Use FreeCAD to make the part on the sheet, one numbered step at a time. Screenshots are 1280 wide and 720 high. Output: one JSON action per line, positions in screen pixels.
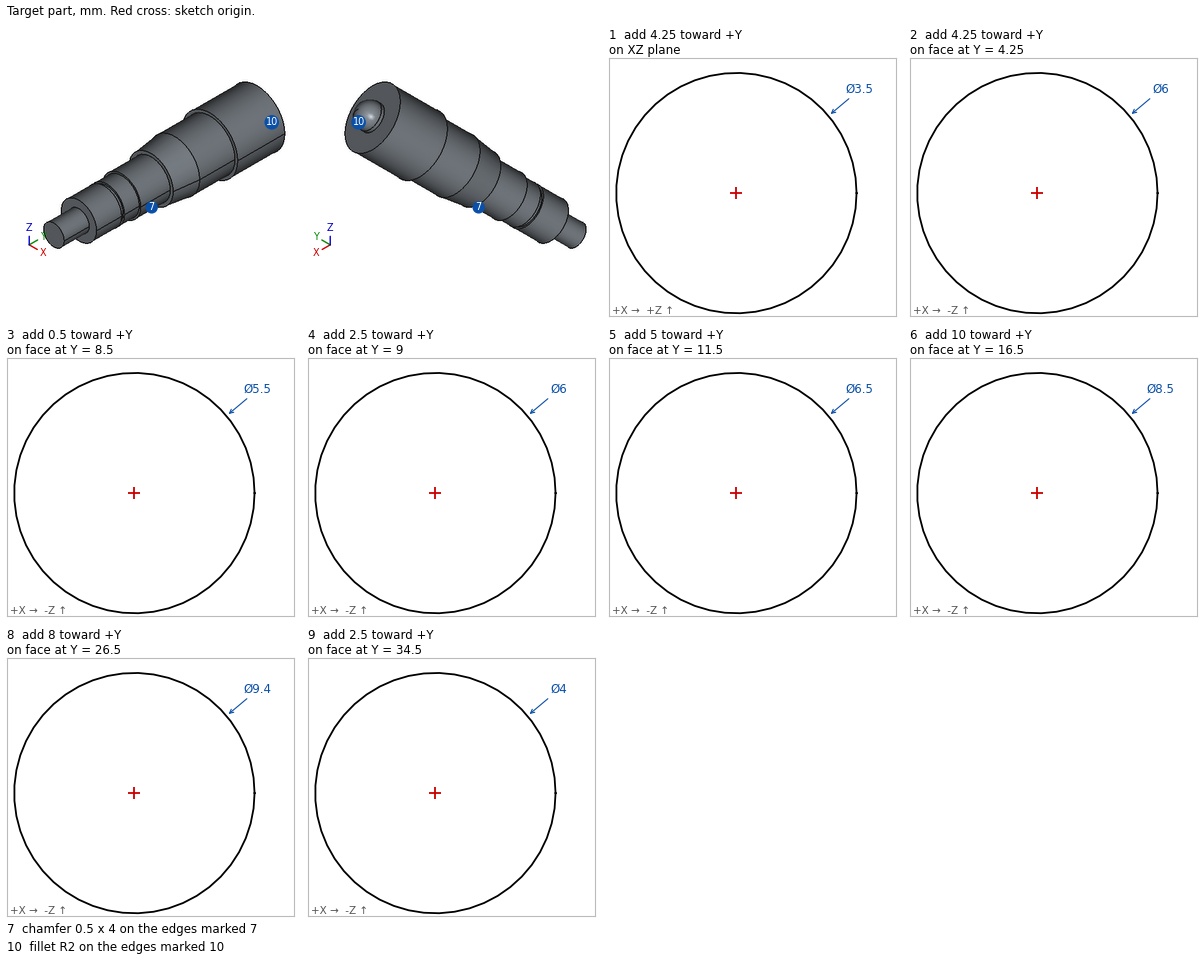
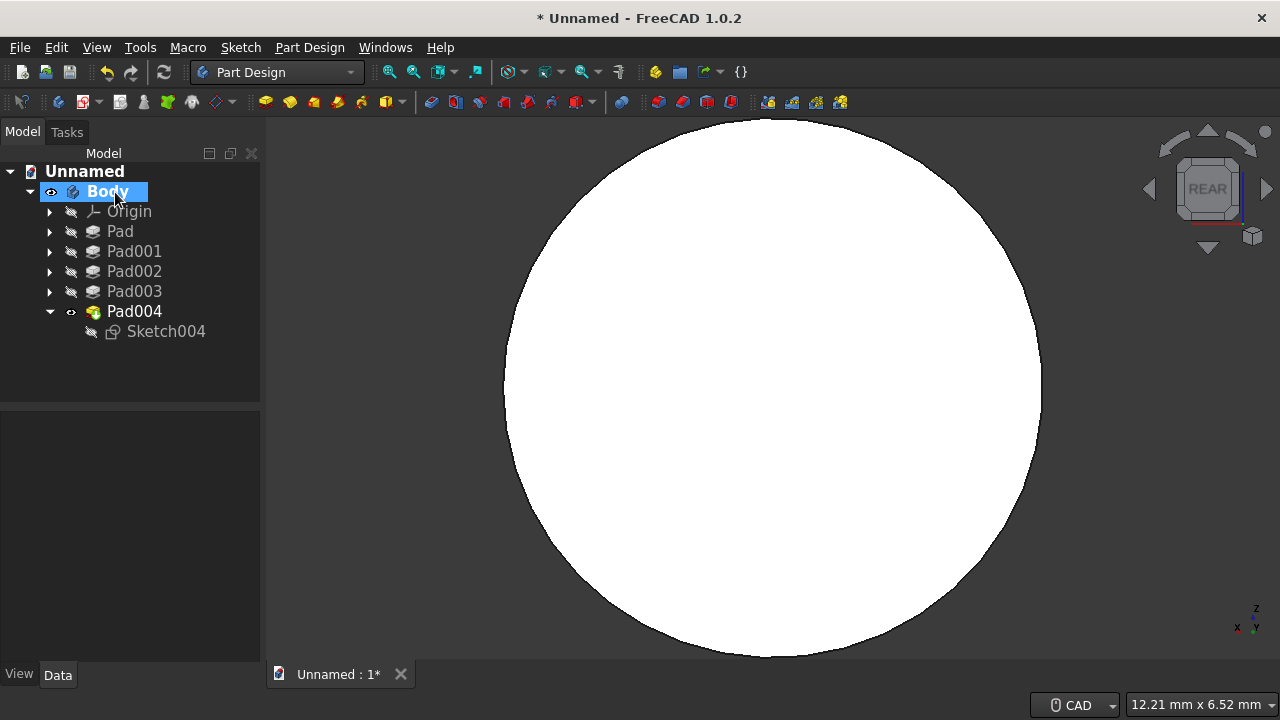
{"action": "left_click", "coordinate": [773, 387]}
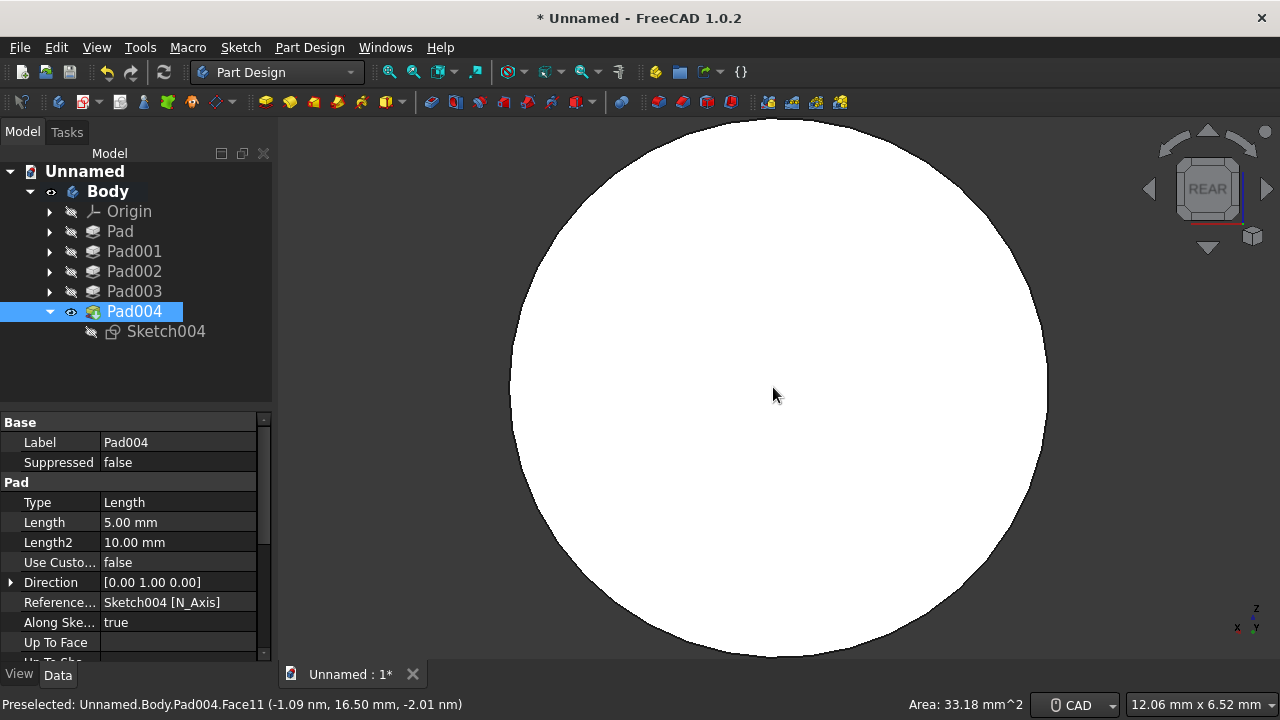
{"action": "left_click", "coordinate": [84, 102]}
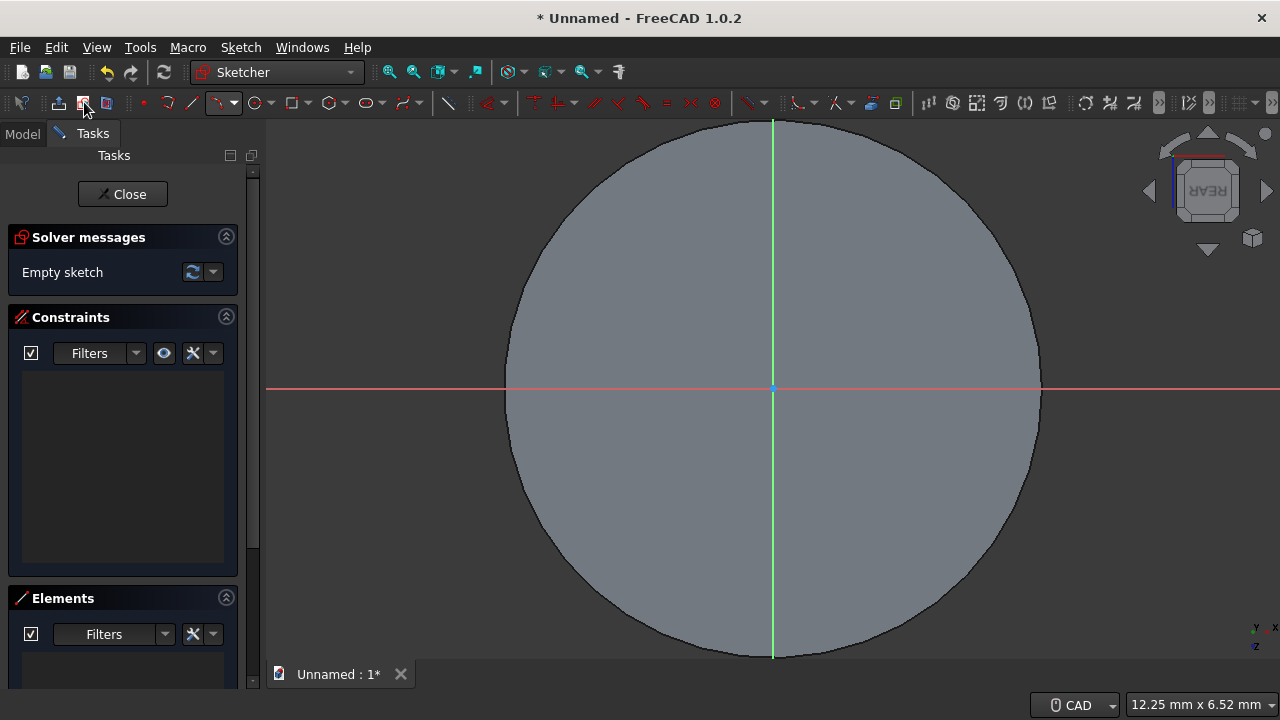
{"action": "scroll", "coordinate": [649, 389], "scroll_direction": "down", "scroll_amount": 4}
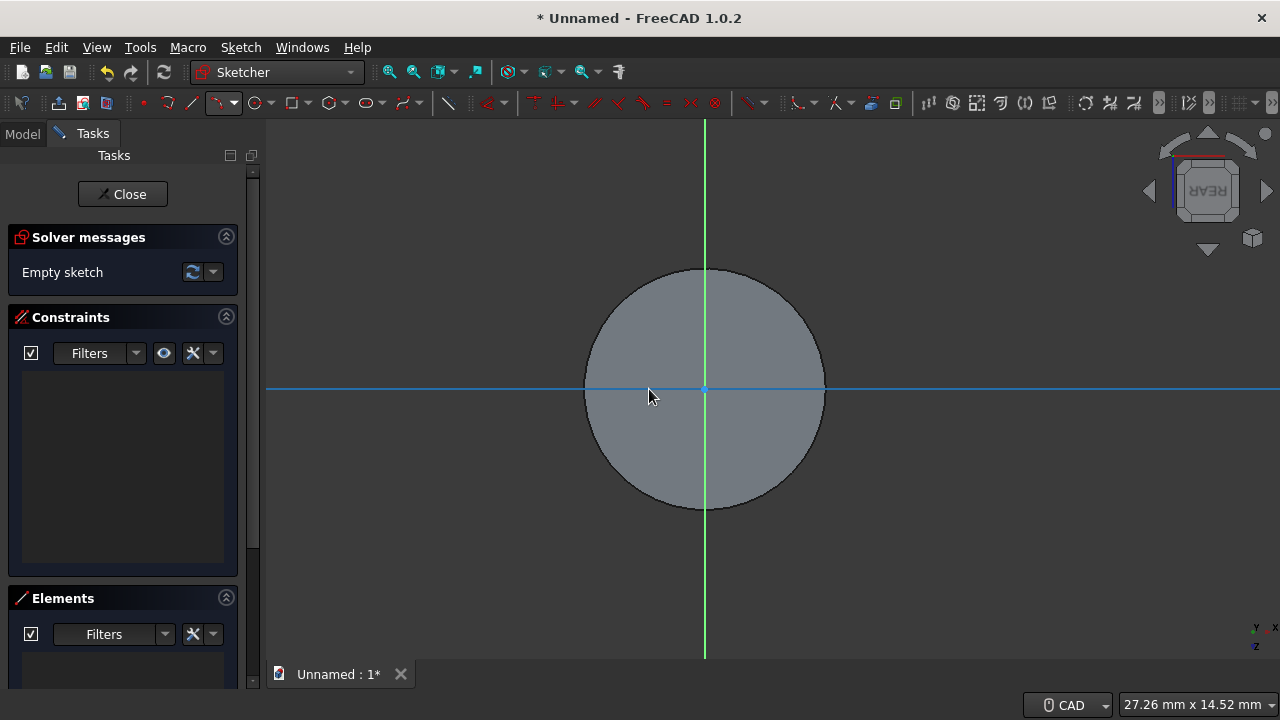
{"action": "key", "text": "g c"}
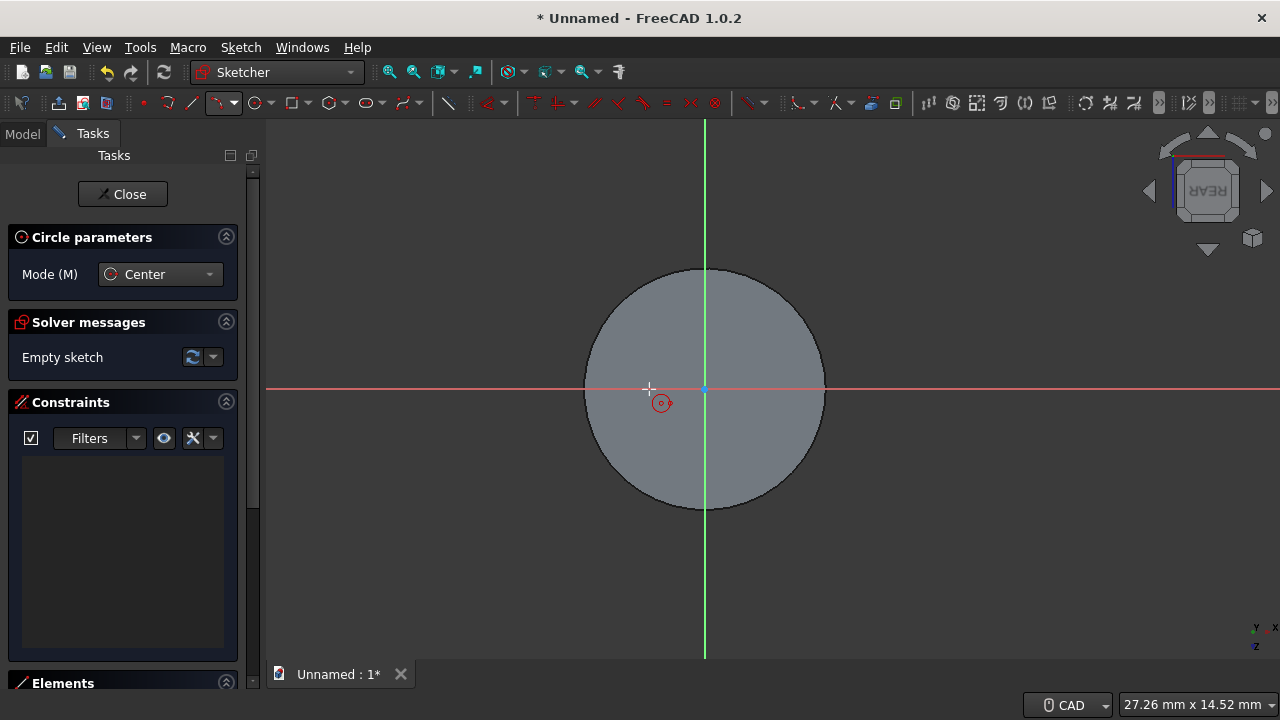
{"action": "left_click", "coordinate": [705, 389]}
{"action": "mouse_move", "coordinate": [817, 278]}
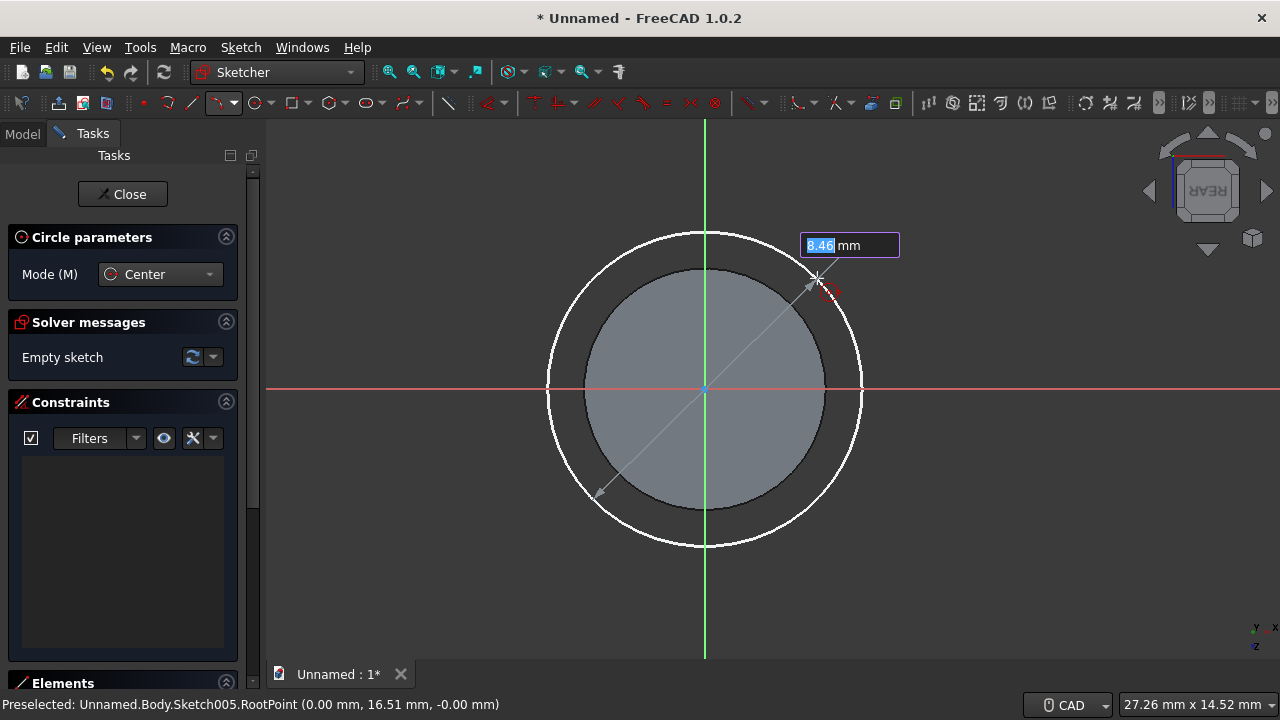
{"action": "type", "text": "8.5"}
{"action": "key", "text": "Return"}
{"action": "key", "text": "Escape"}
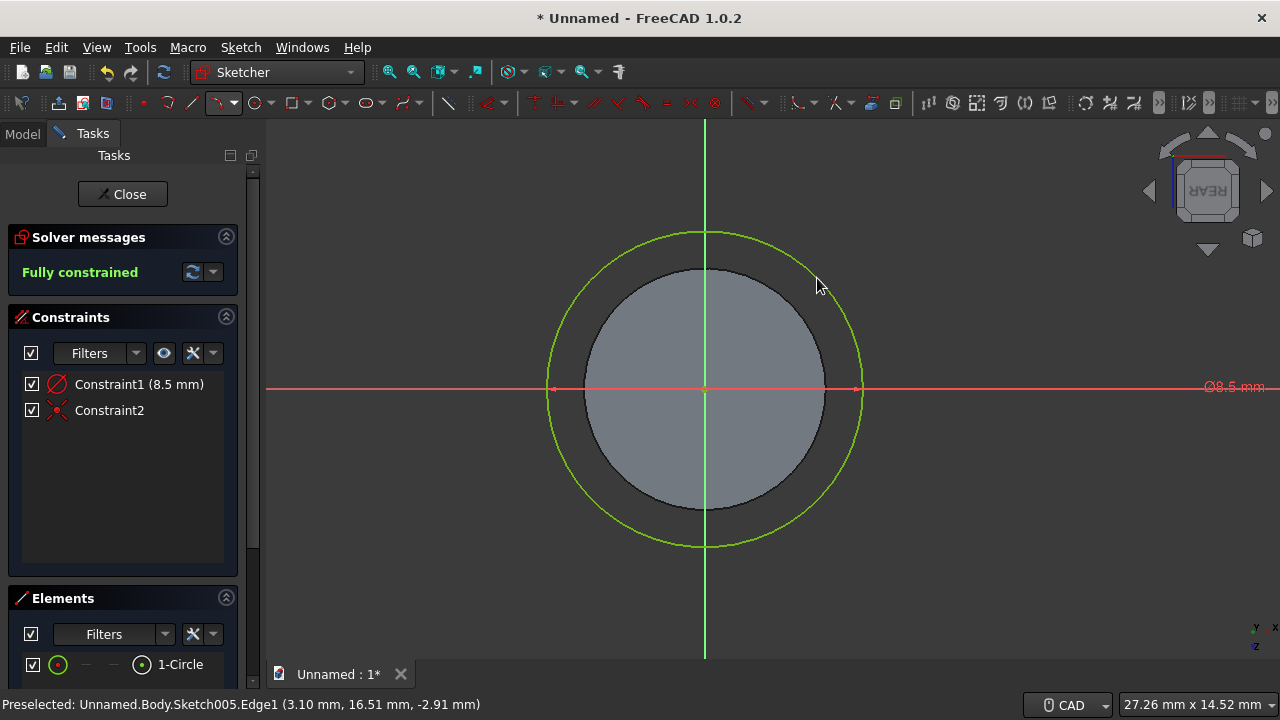
{"action": "left_click", "coordinate": [123, 194]}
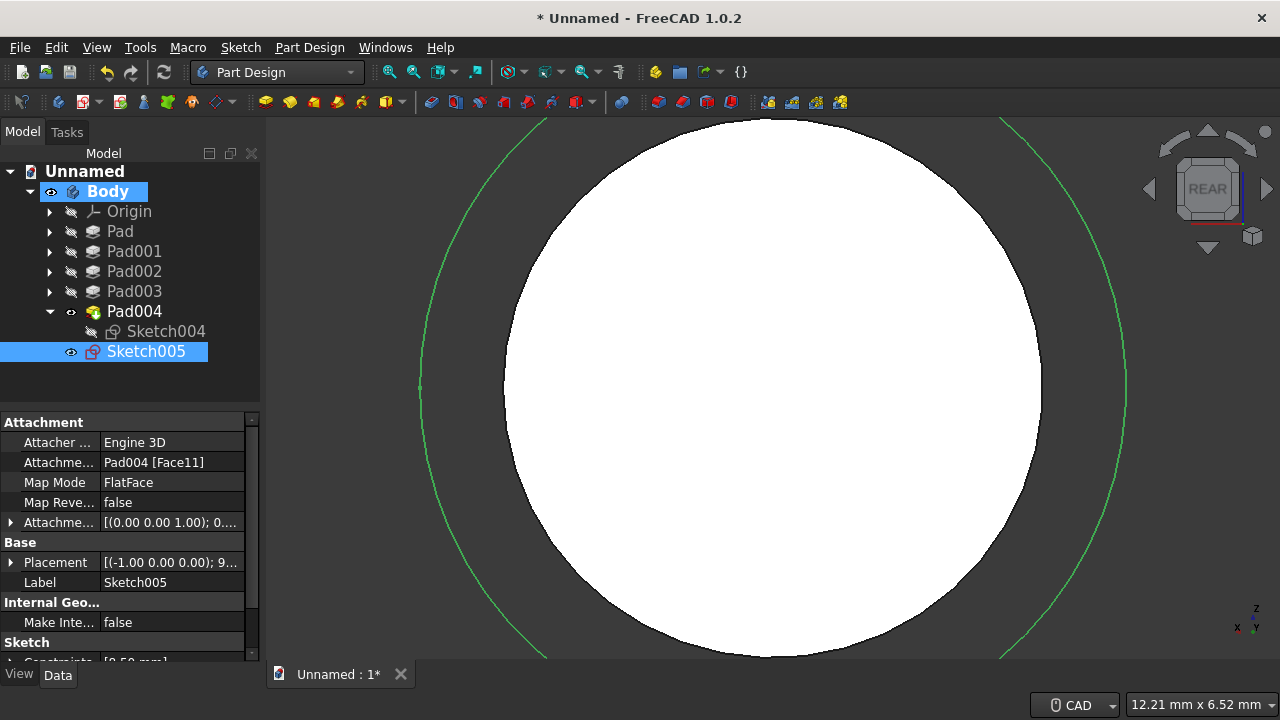
{"action": "left_click", "coordinate": [266, 102]}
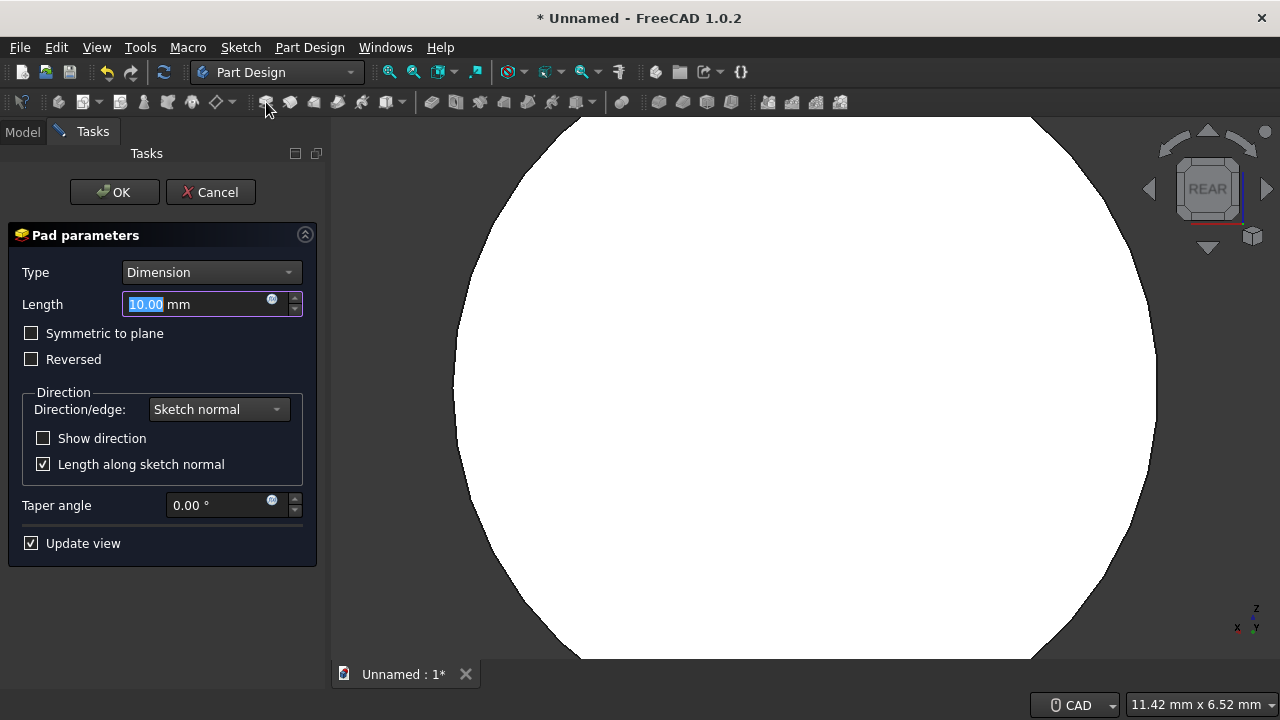
{"action": "type", "text": "10"}
{"action": "key", "text": "Tab"}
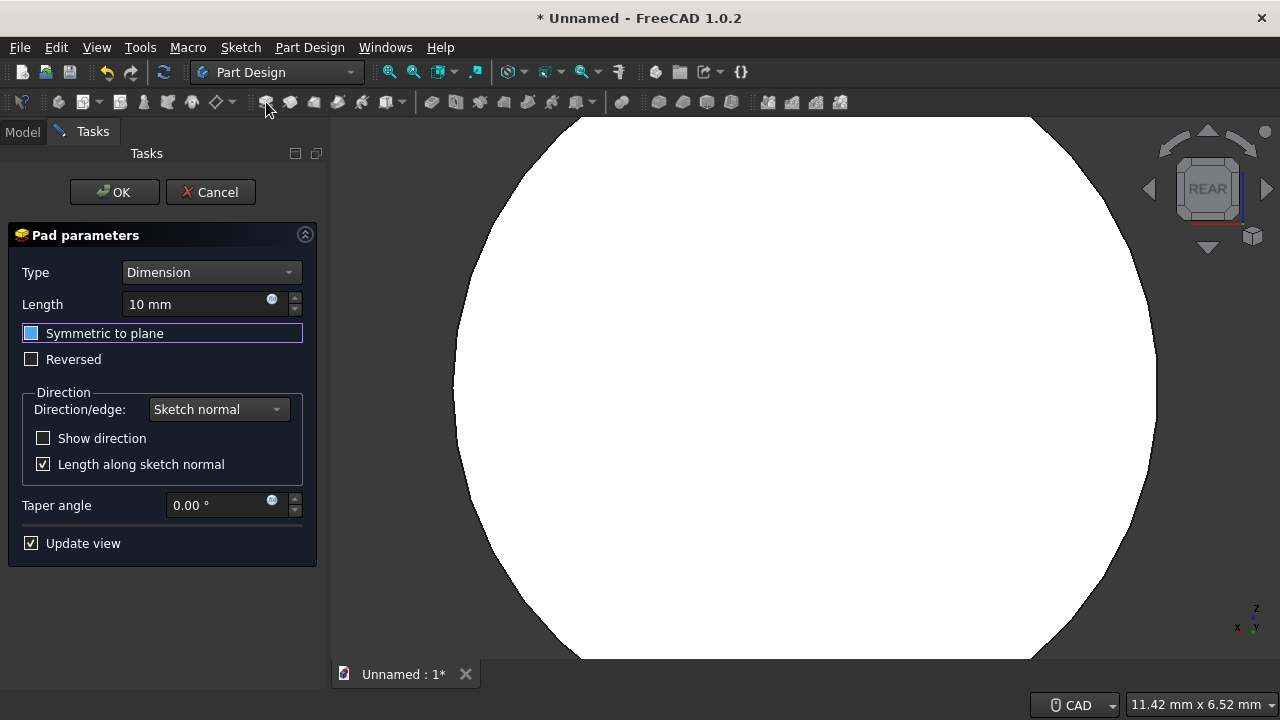
{"action": "left_click", "coordinate": [115, 192]}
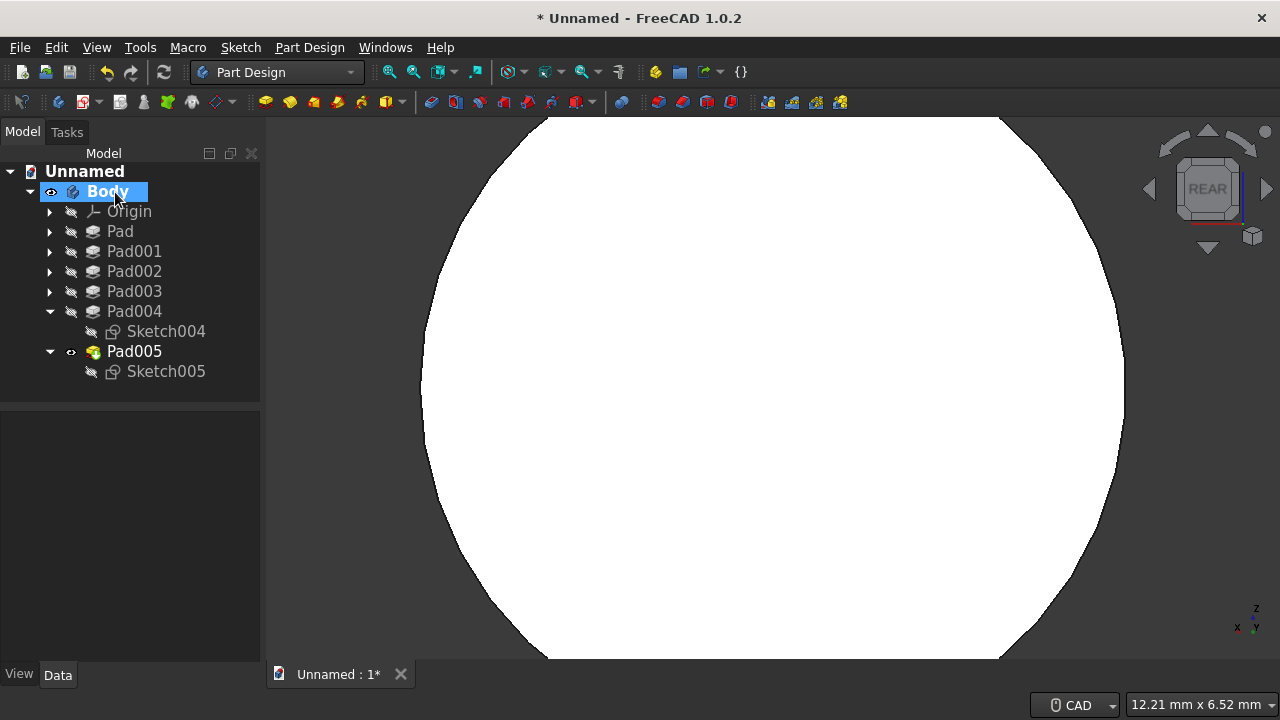
{"action": "key", "text": "v f"}